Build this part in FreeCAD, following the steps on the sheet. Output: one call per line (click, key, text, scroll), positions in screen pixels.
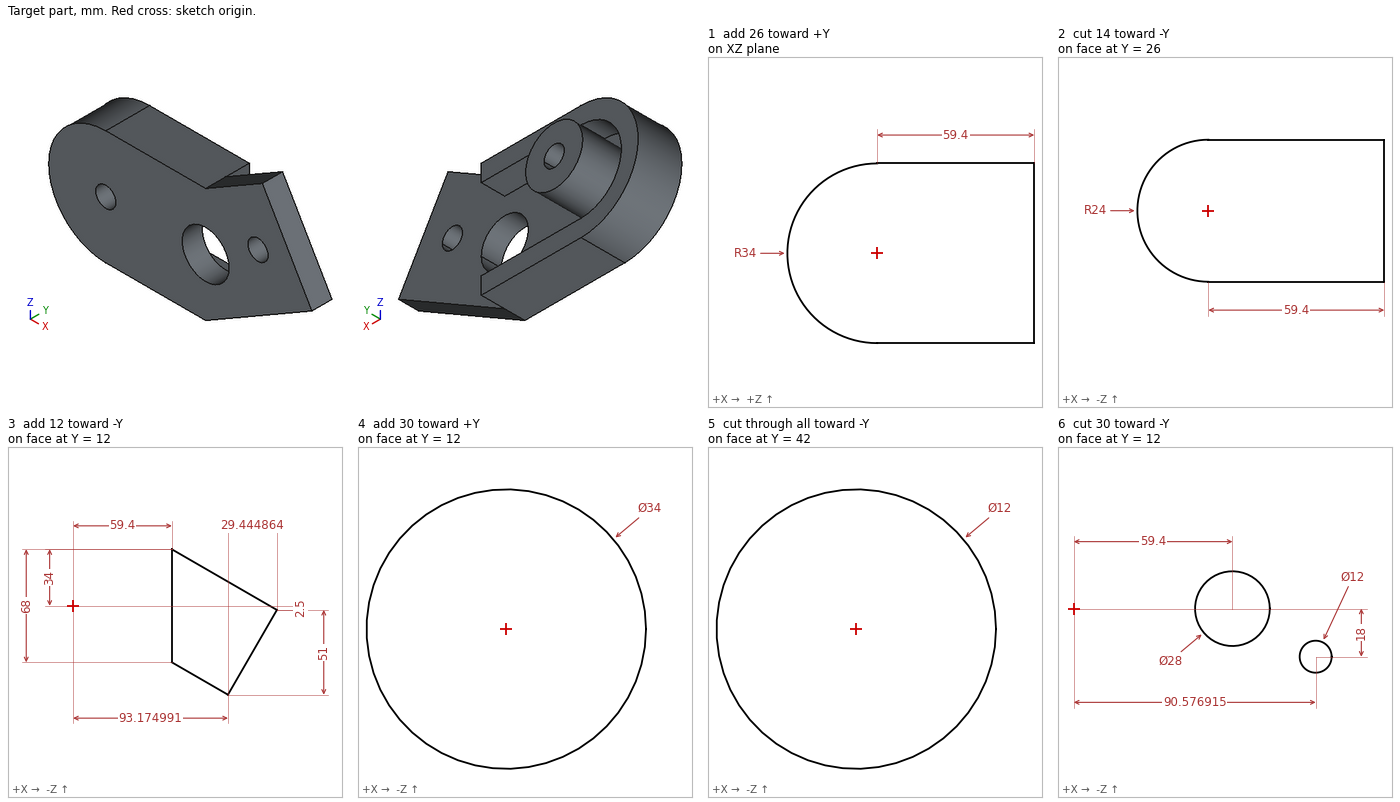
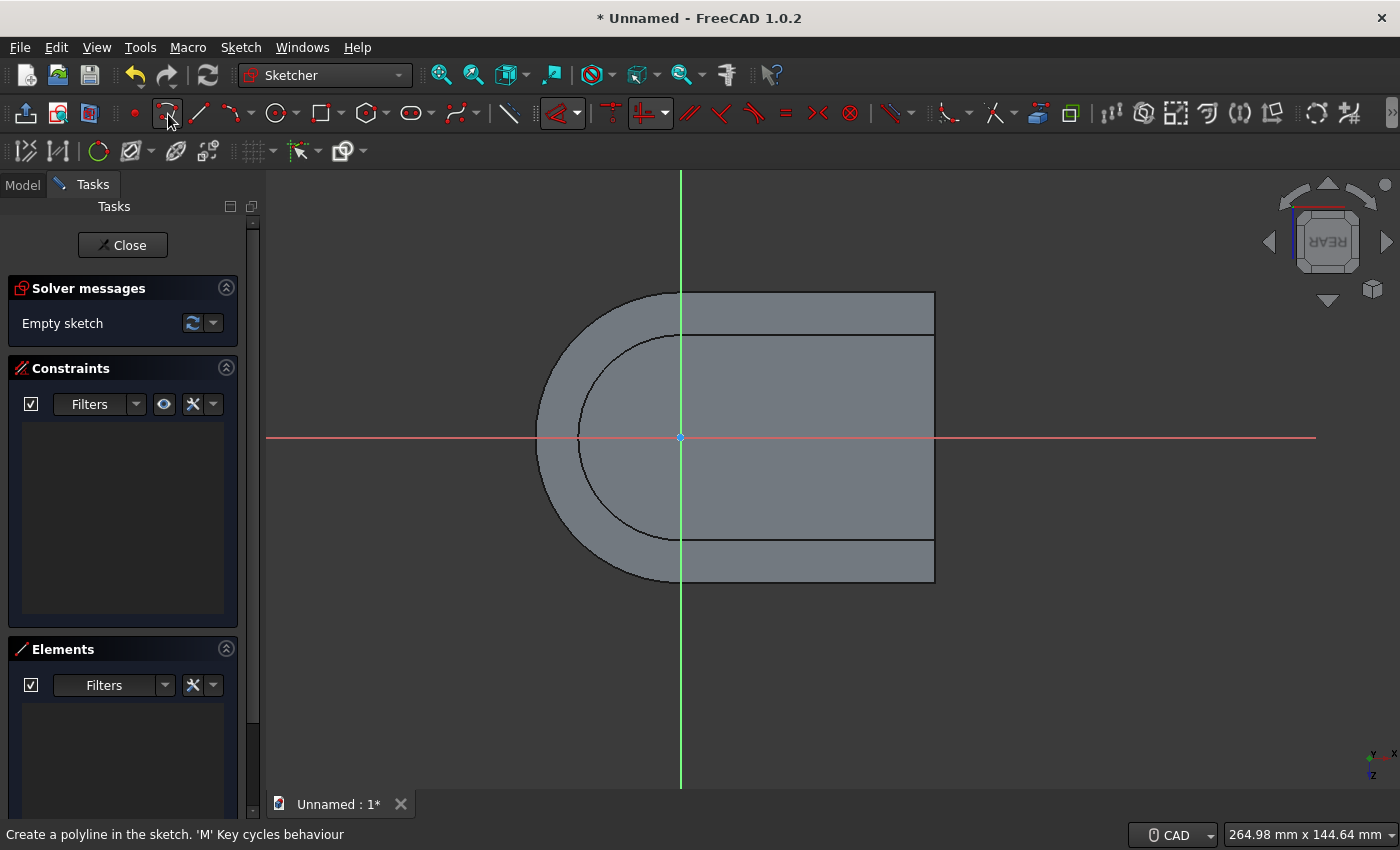
click(935, 292)
click(935, 583)
click(1080, 667)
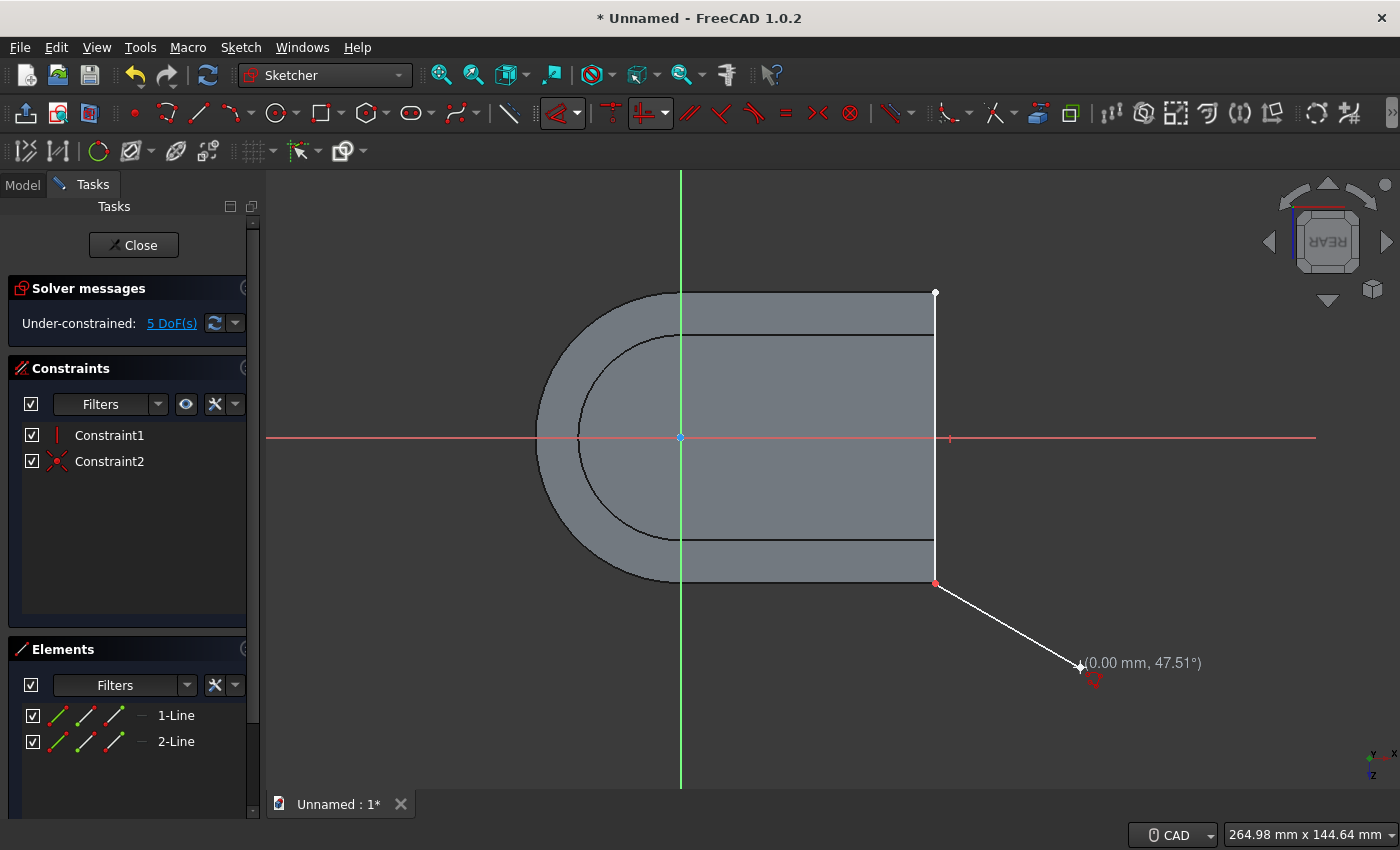
scroll(1206, 448, up, 2)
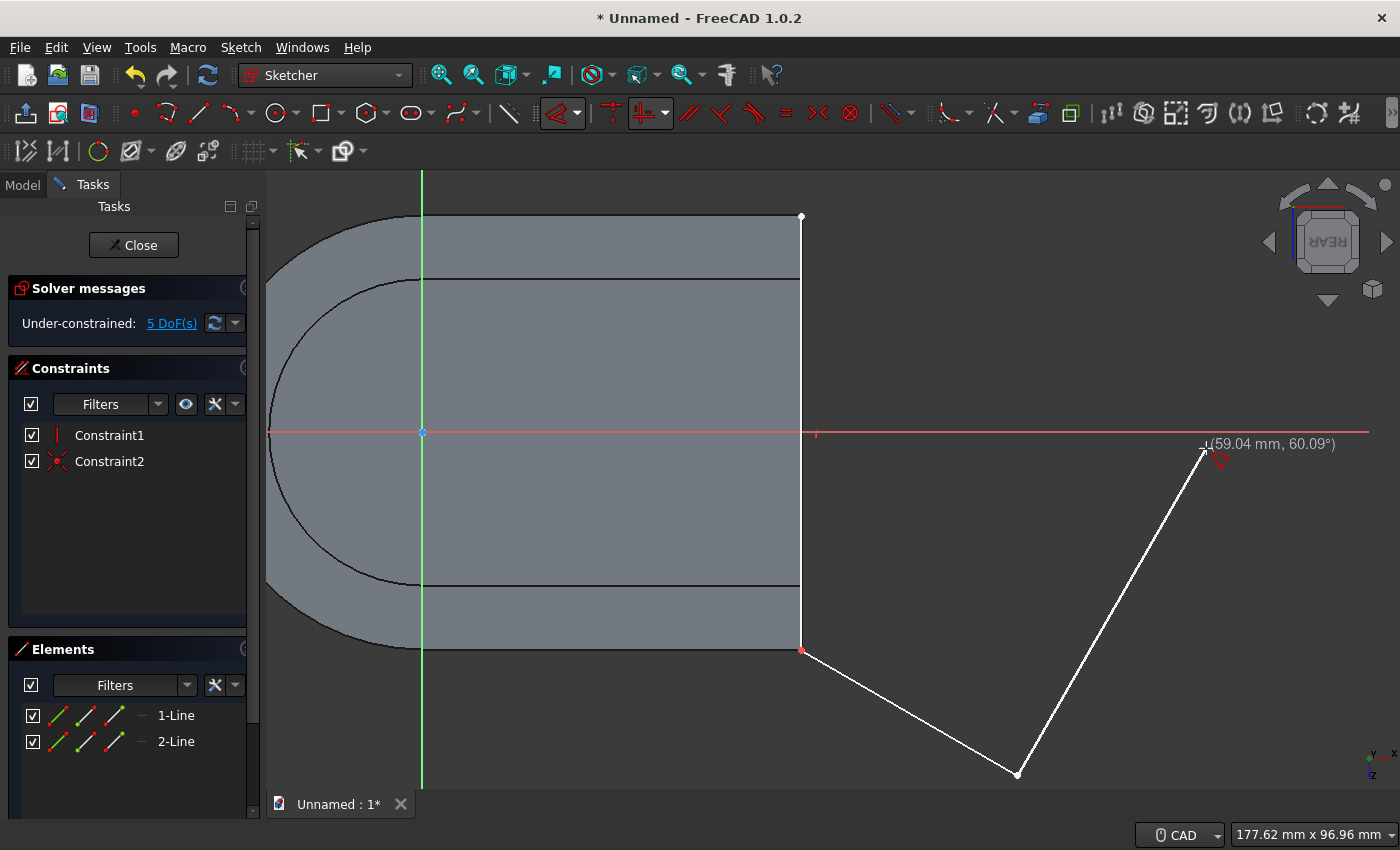
click(1205, 448)
click(801, 217)
key(Escape)
key(Escape)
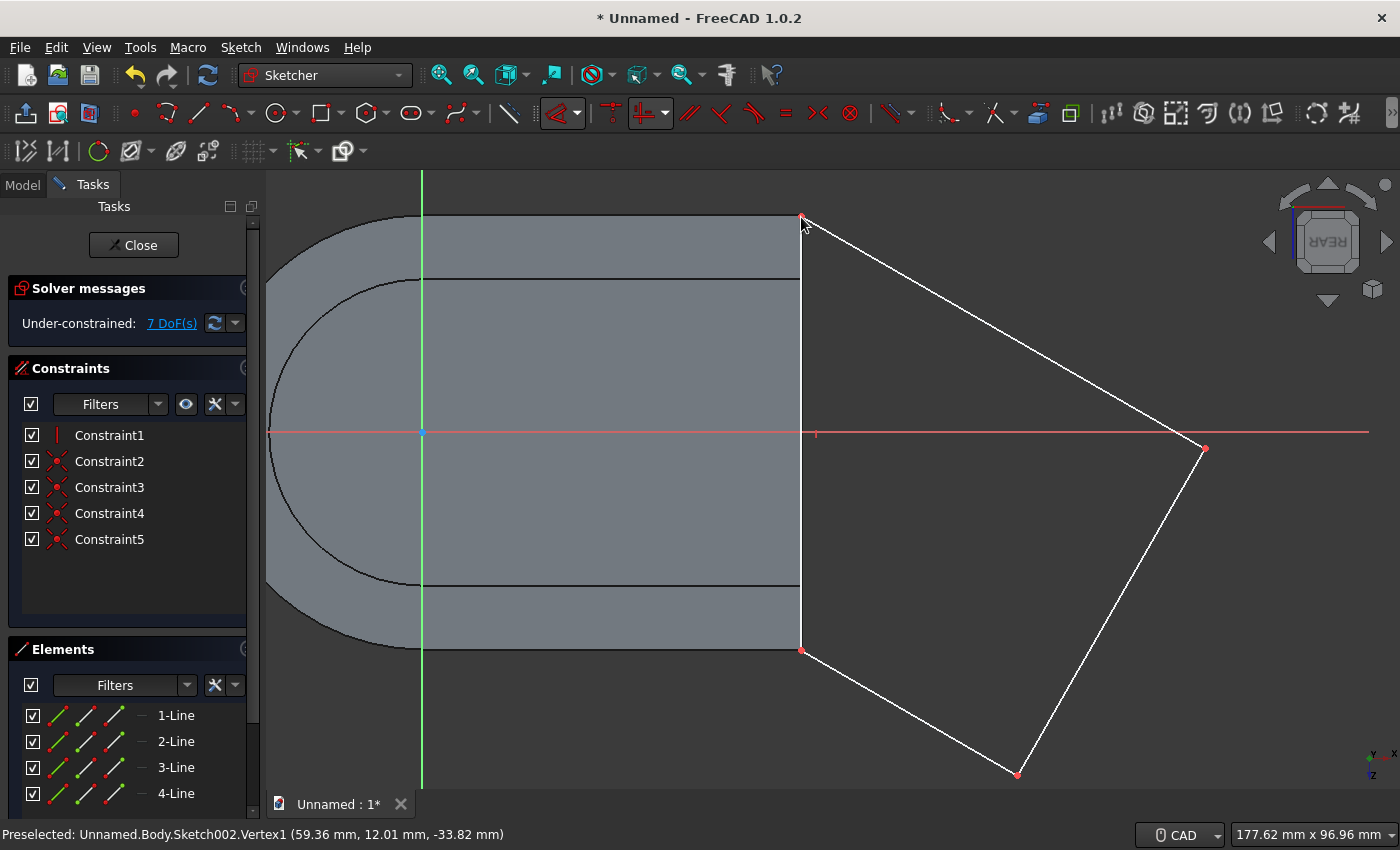
click(801, 347)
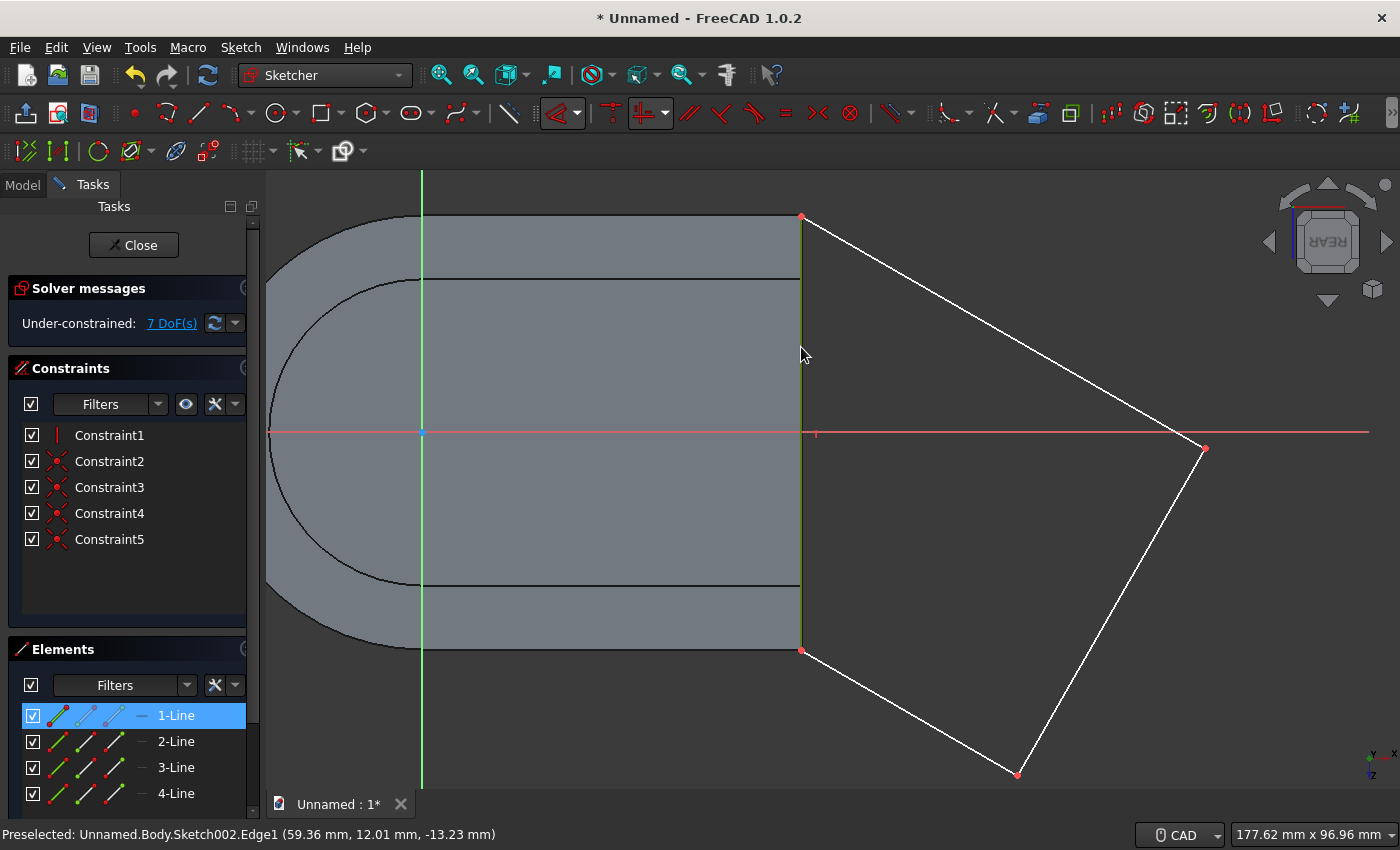
key(i)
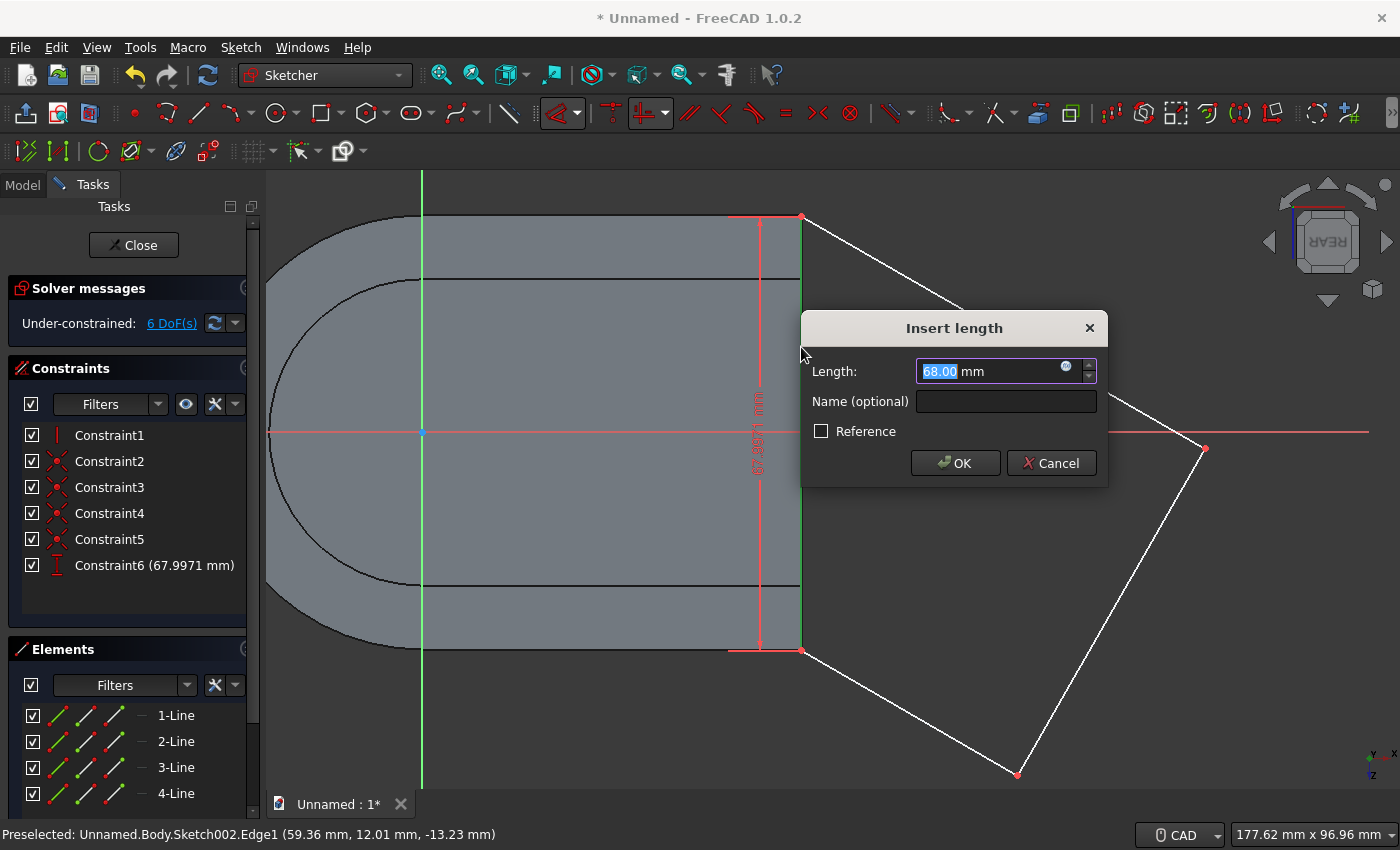
text(68)
key(Return)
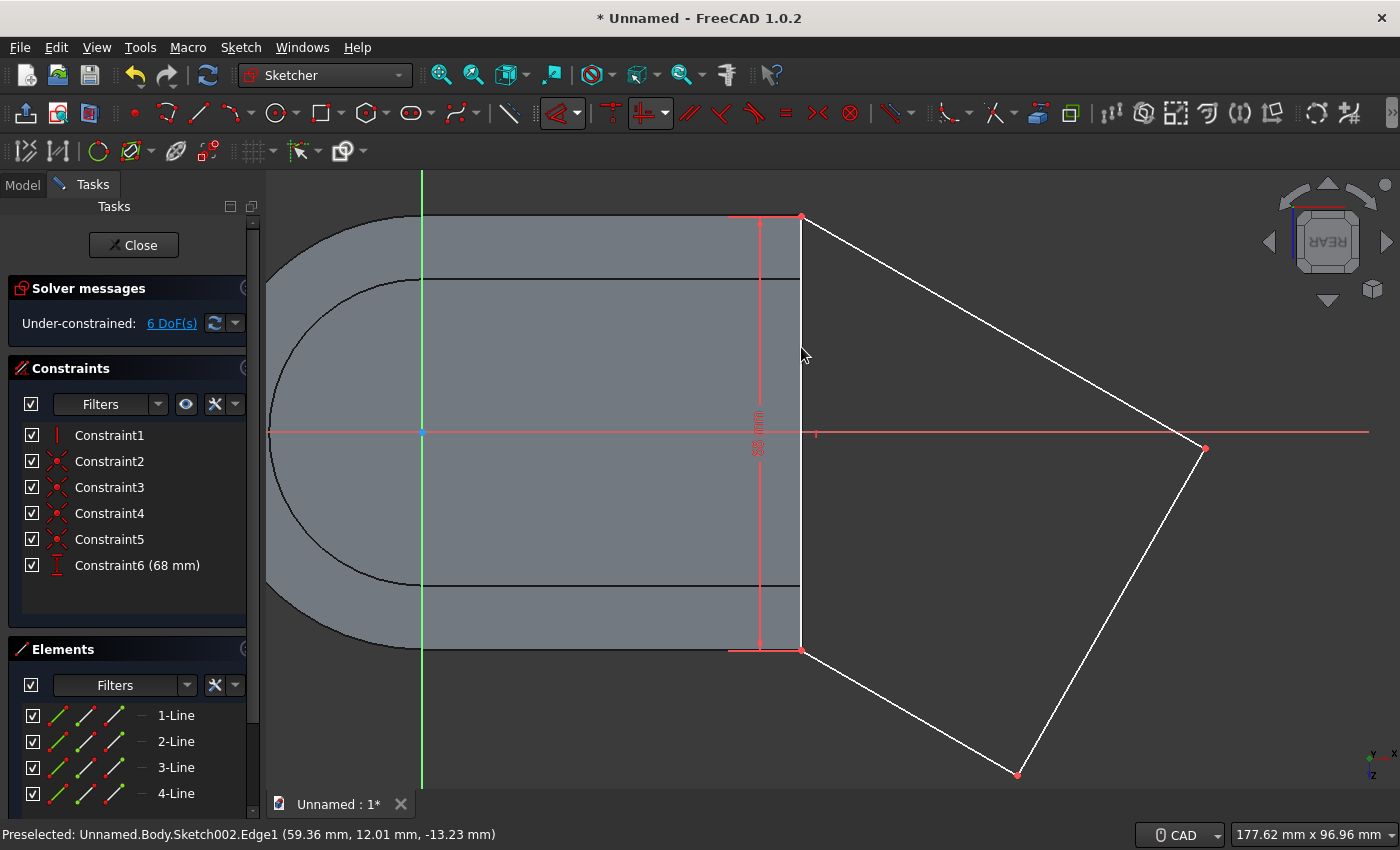
click(801, 217)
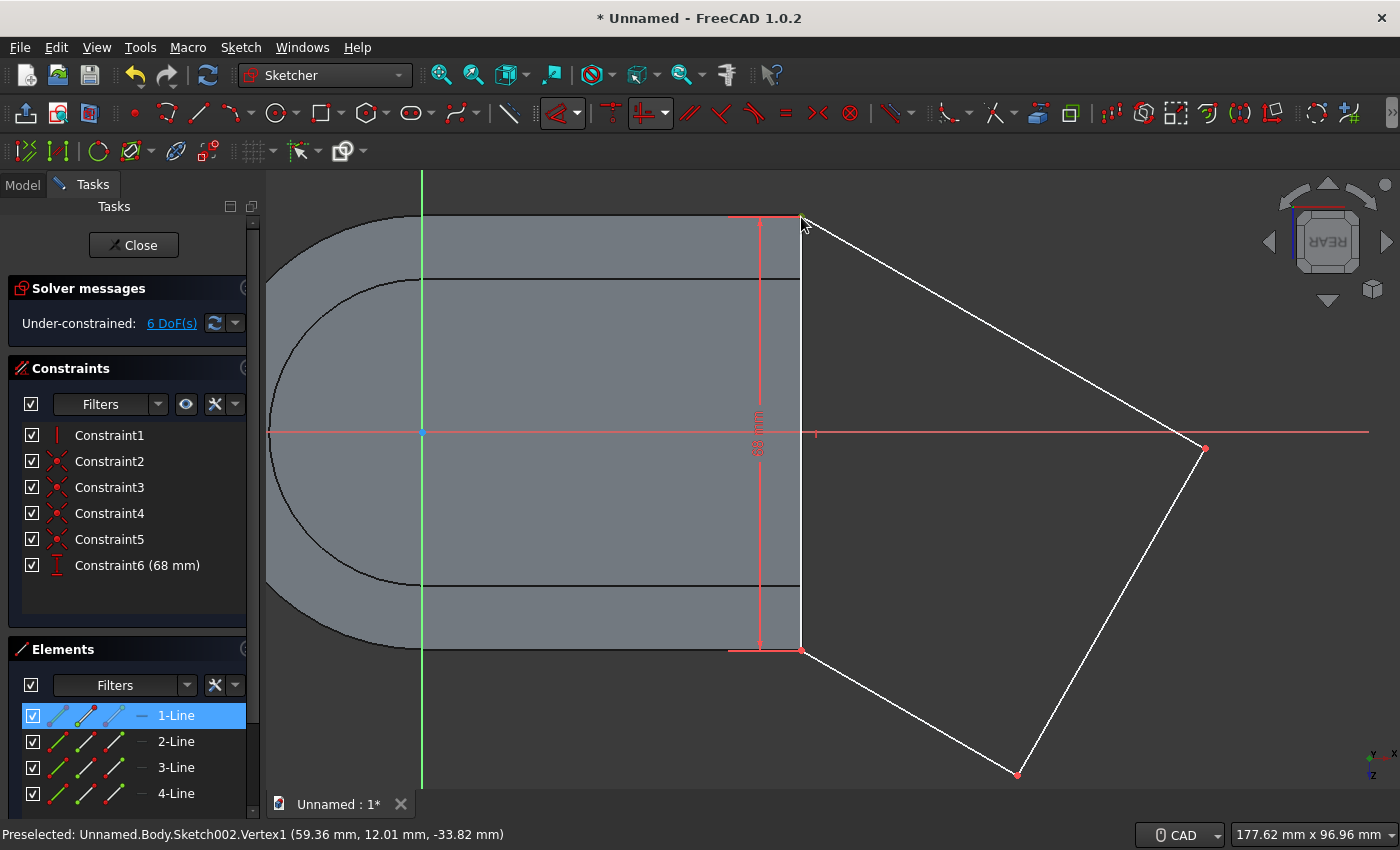
key(i)